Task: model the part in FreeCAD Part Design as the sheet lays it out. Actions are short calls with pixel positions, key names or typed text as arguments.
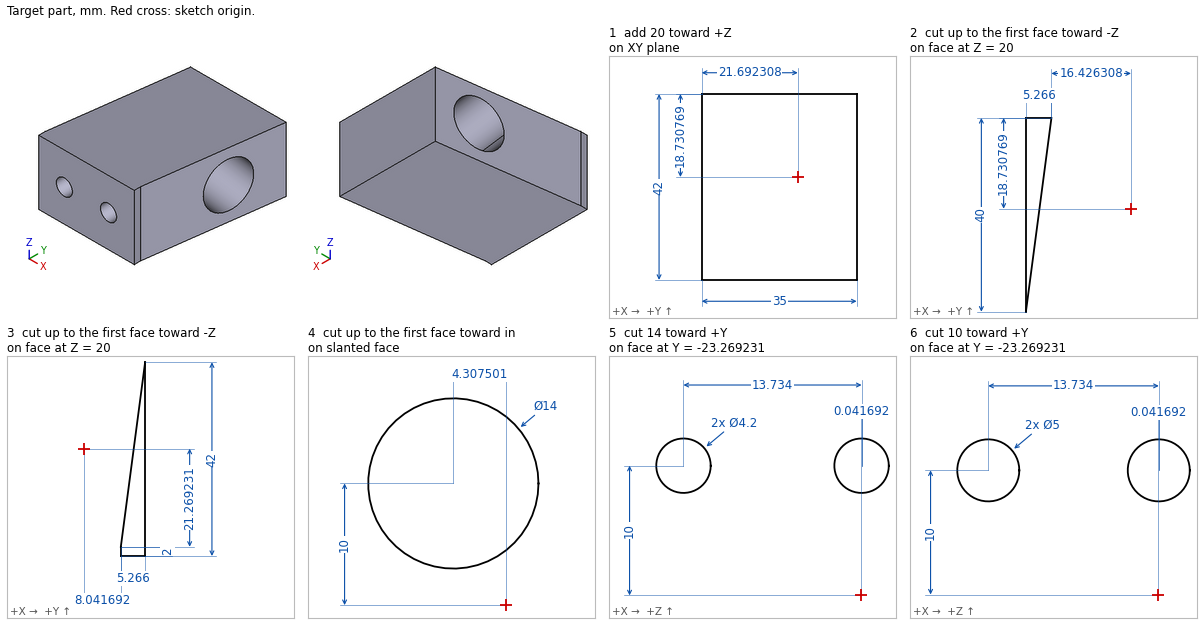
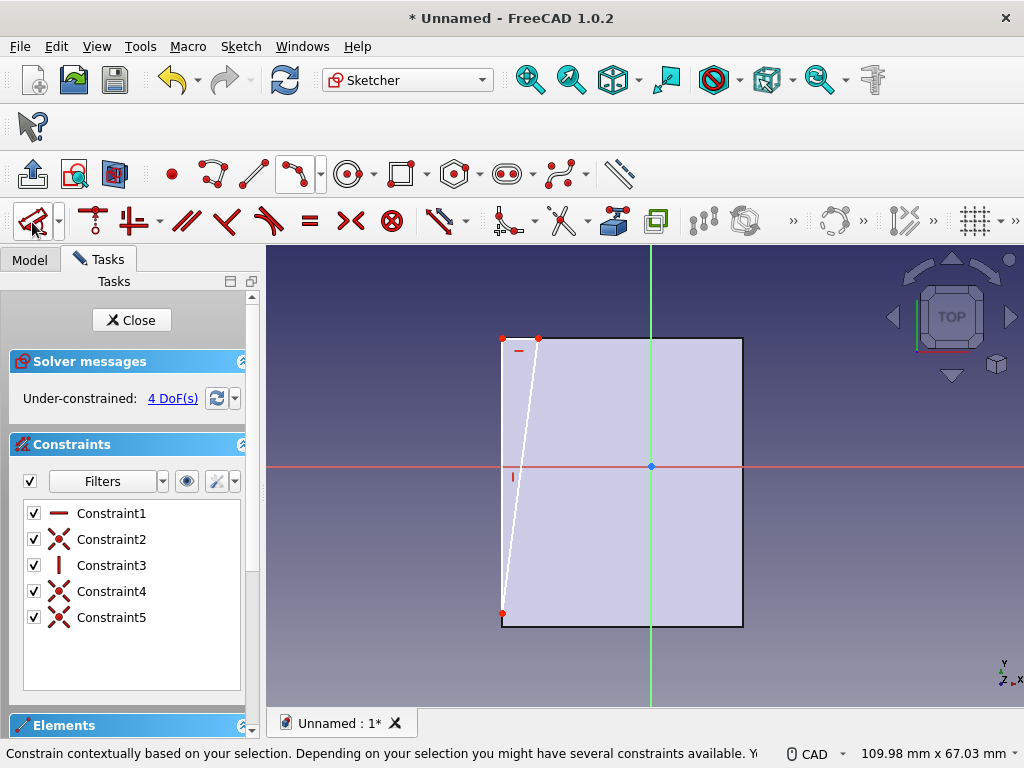
click(502, 421)
click(468, 413)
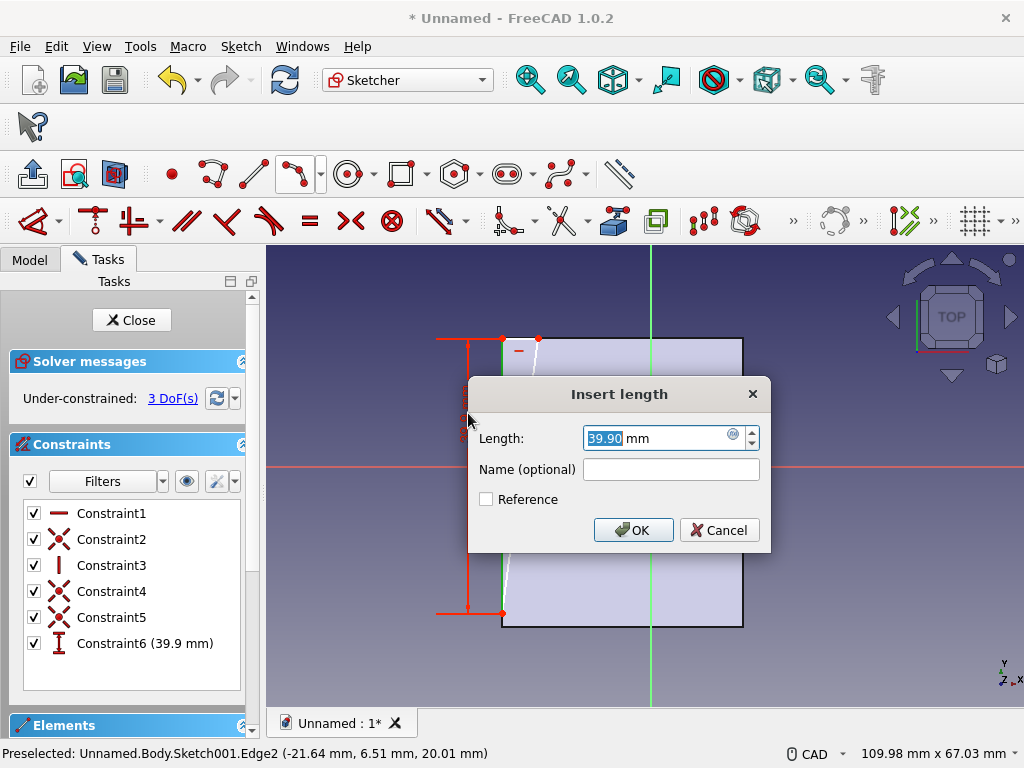
text(40)
key(Return)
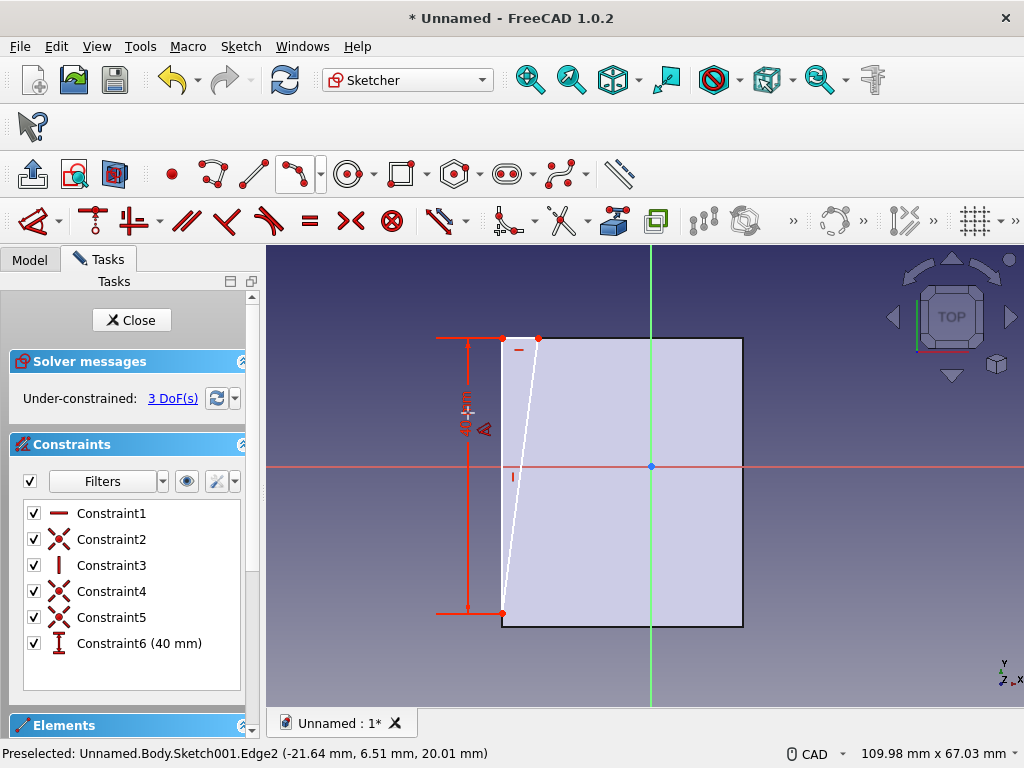
scroll(527, 338, up, 2)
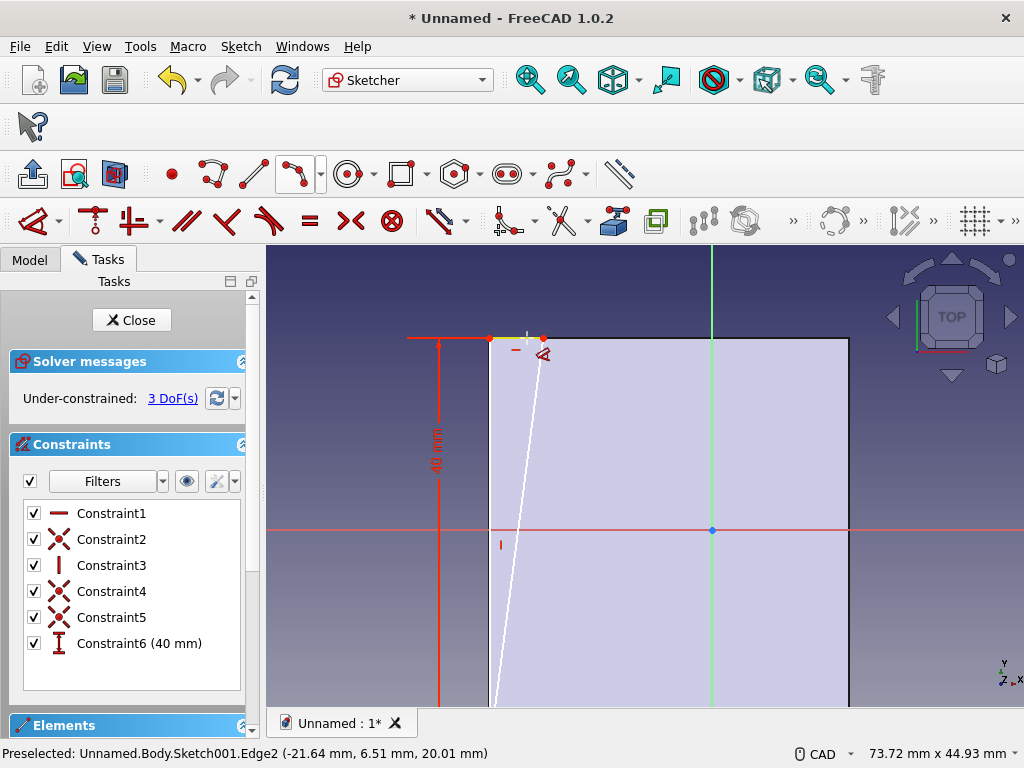
click(527, 338)
click(516, 304)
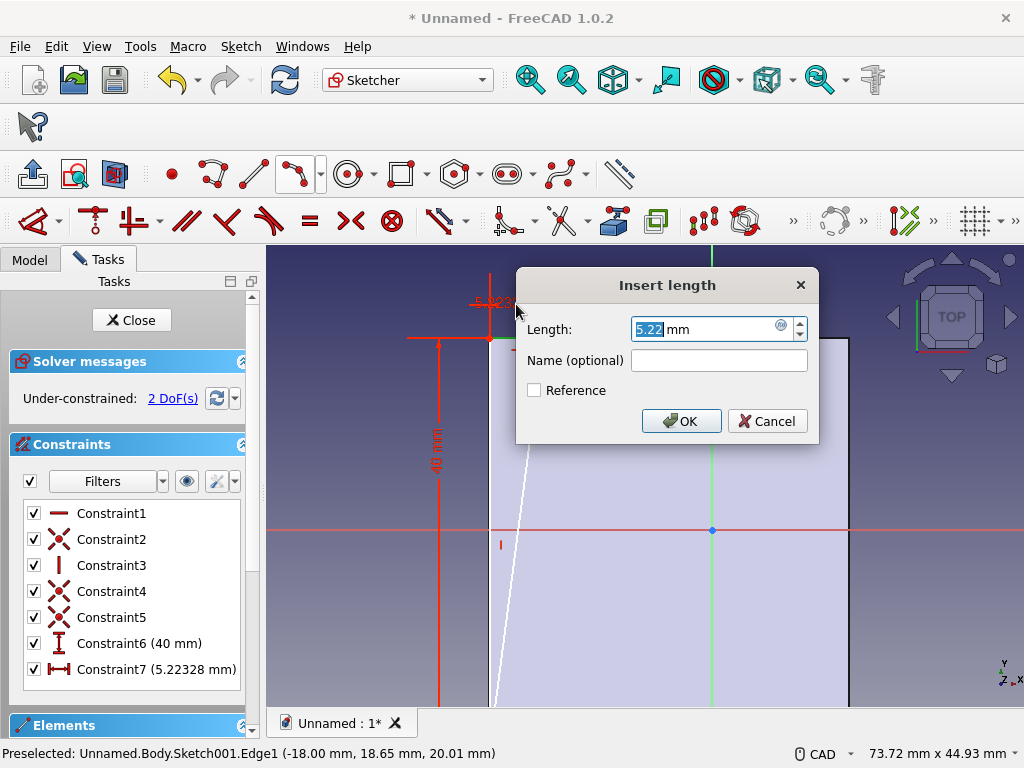
text(5.266)
key(Return)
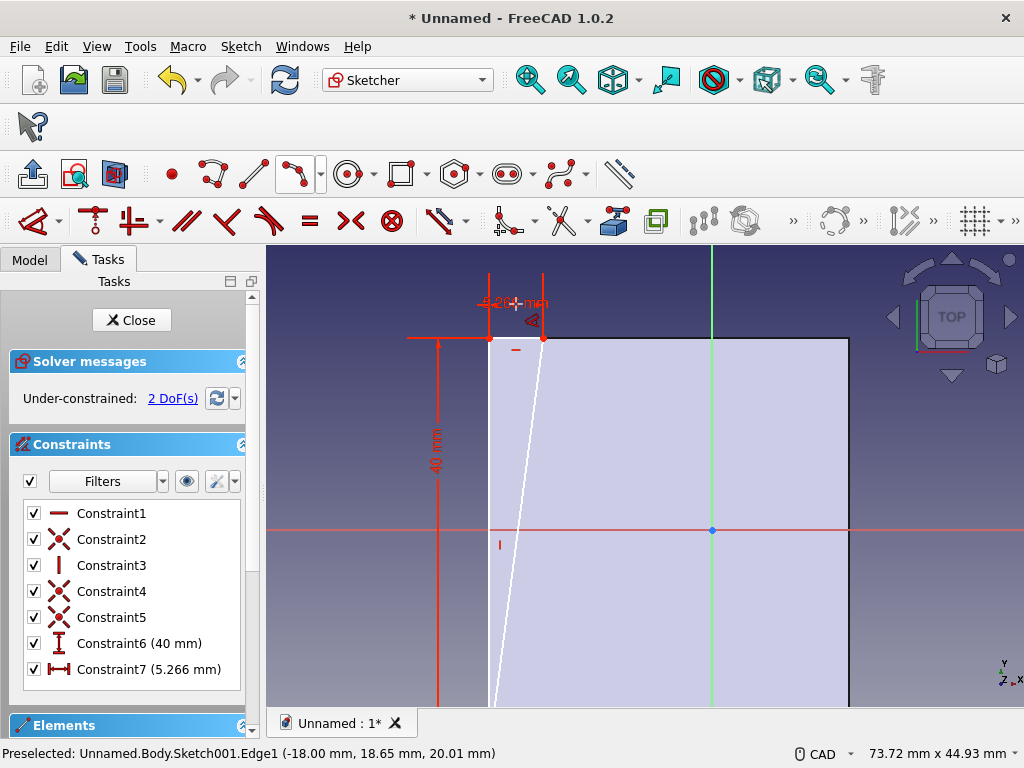
click(543, 338)
click(628, 304)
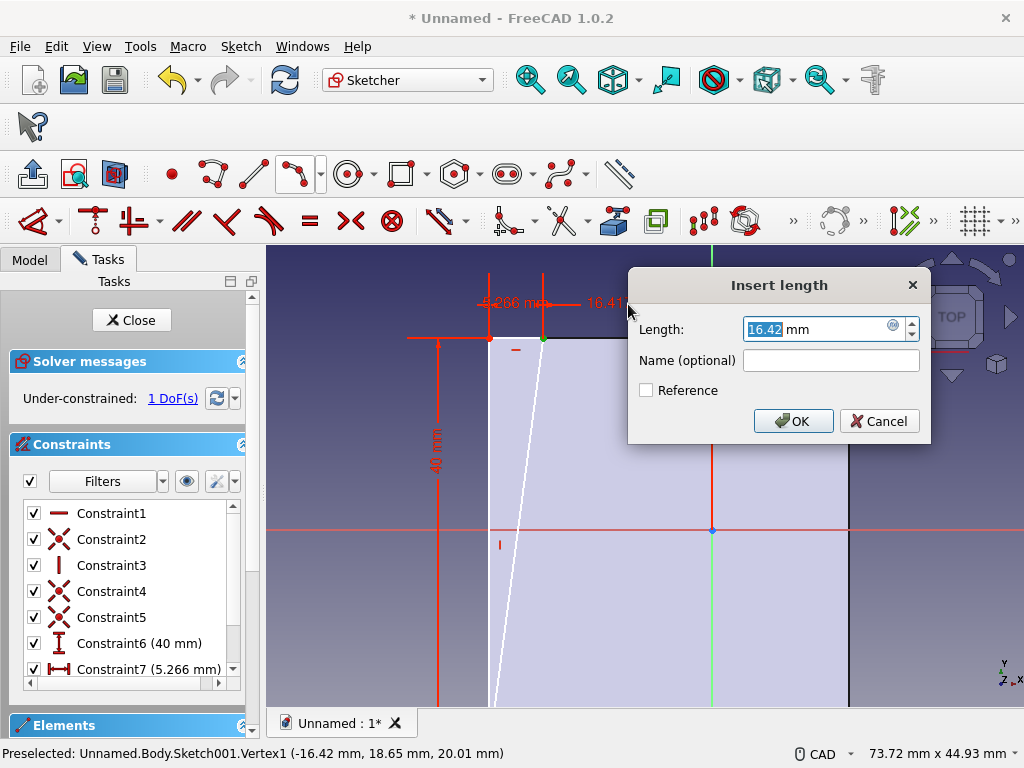
text(16.426308)
key(Return)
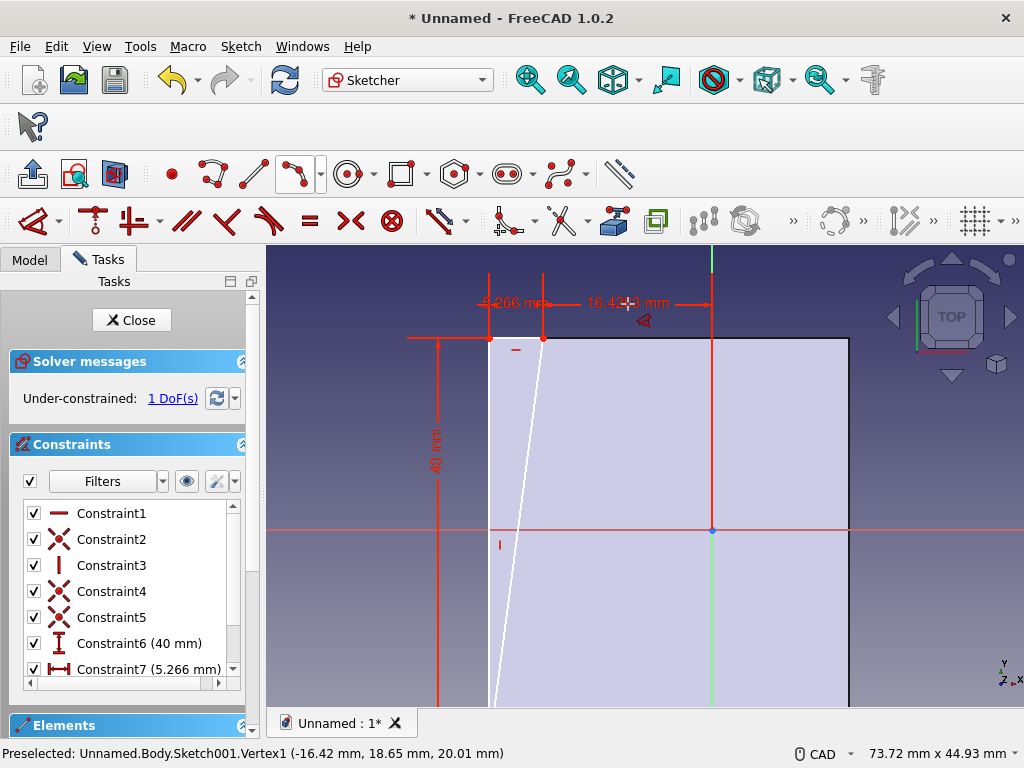
click(543, 338)
click(746, 434)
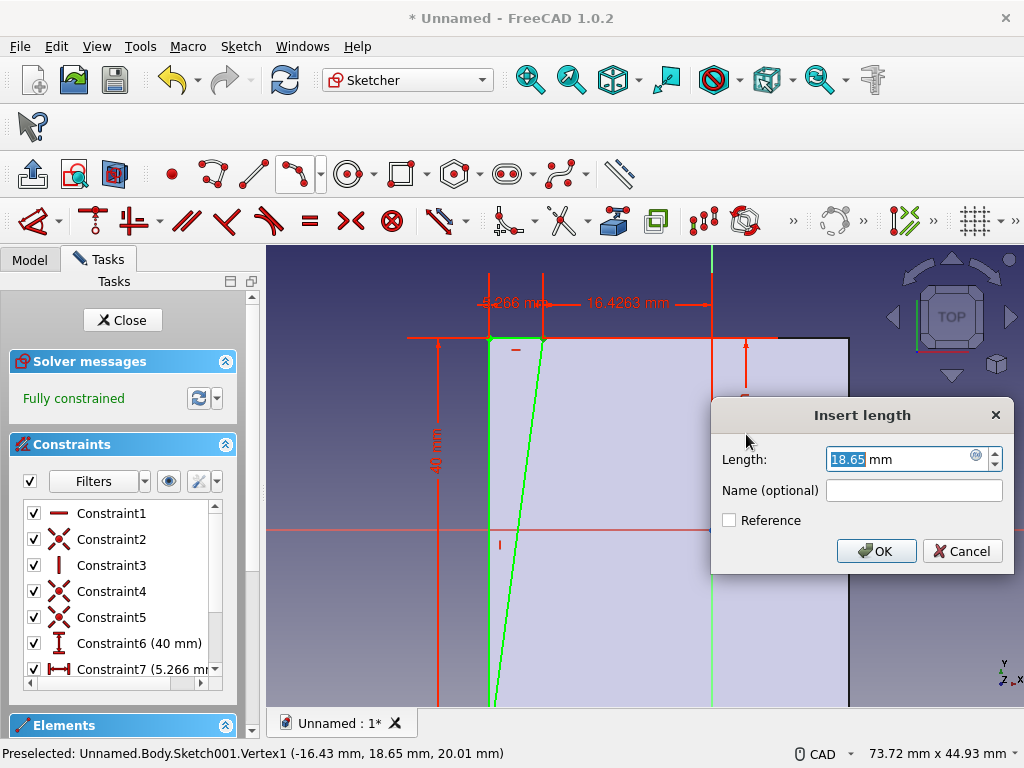
text(18.730769)
key(Return)
key(Escape)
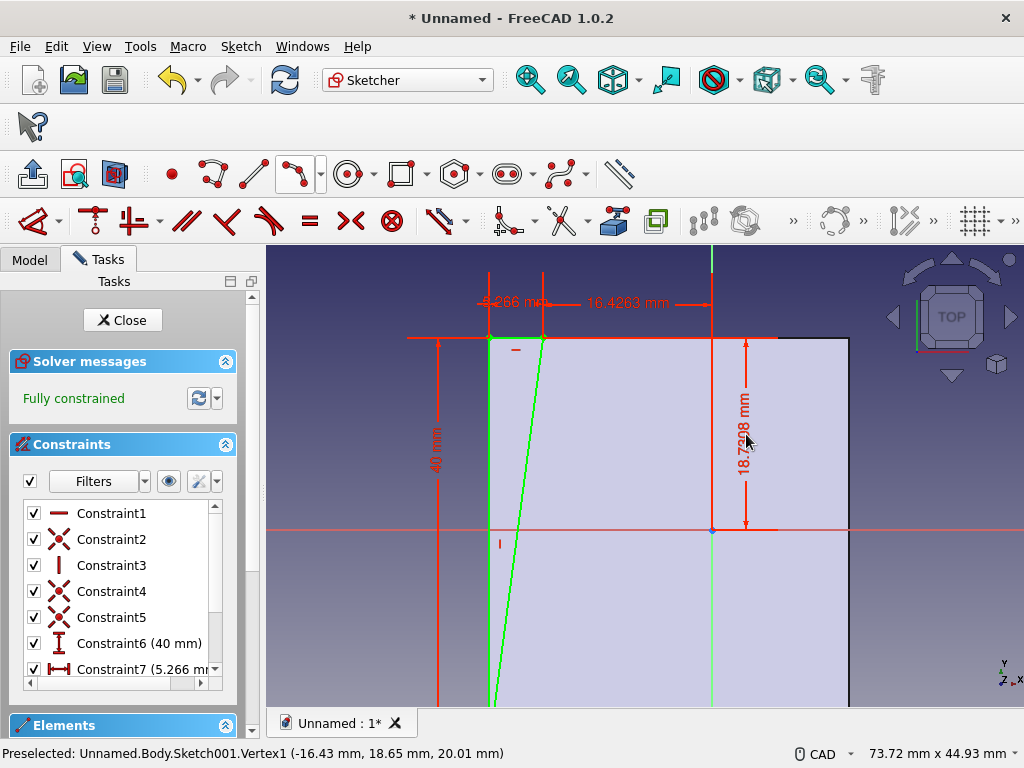
click(123, 320)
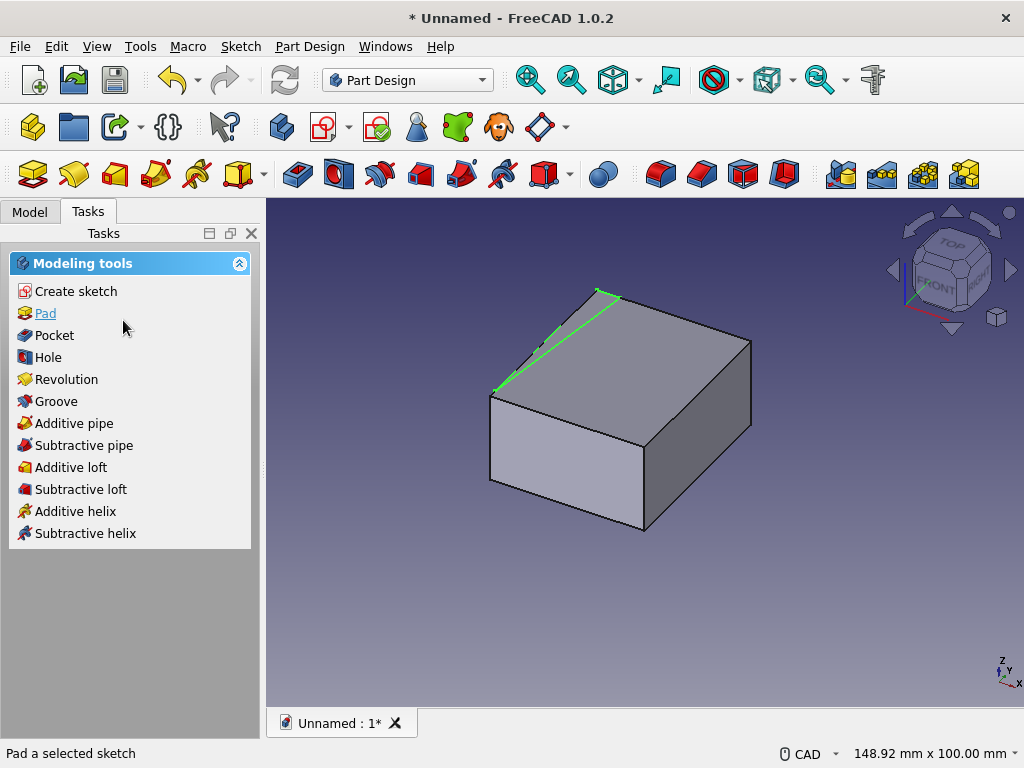
click(298, 174)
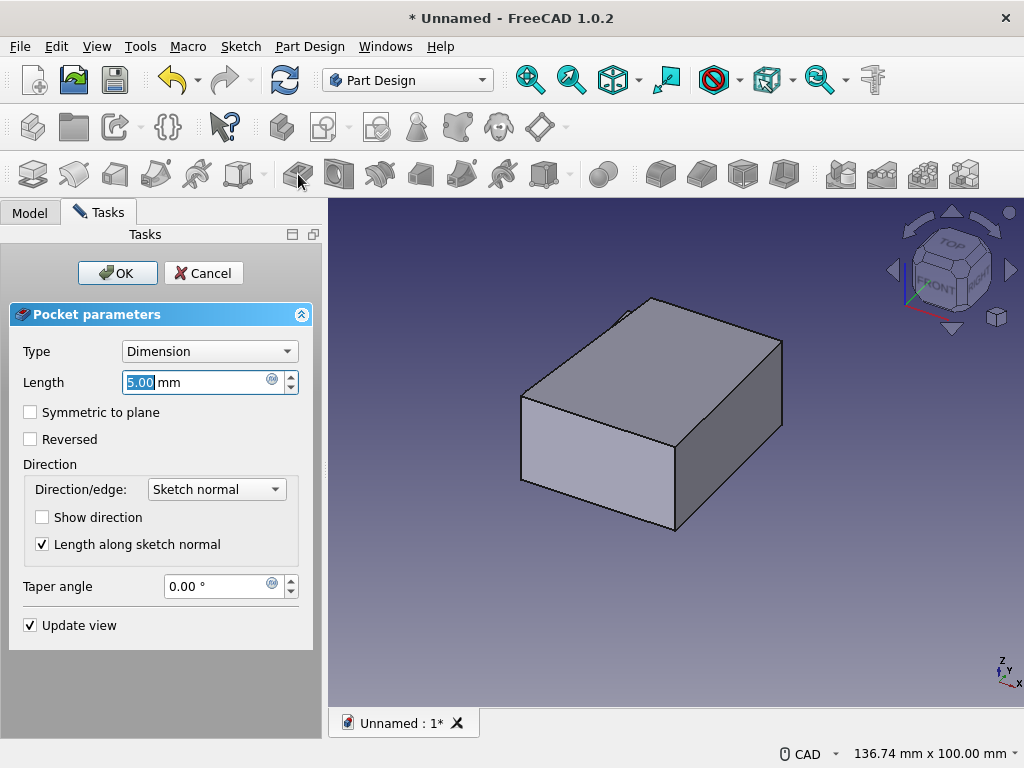
click(210, 352)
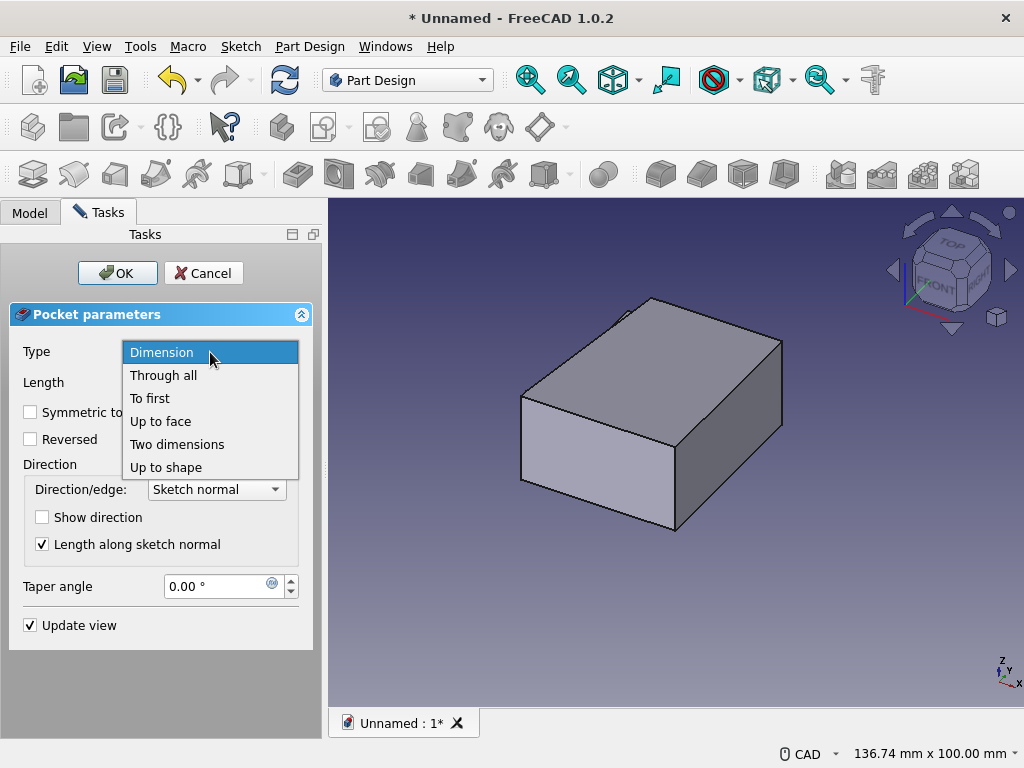
click(208, 398)